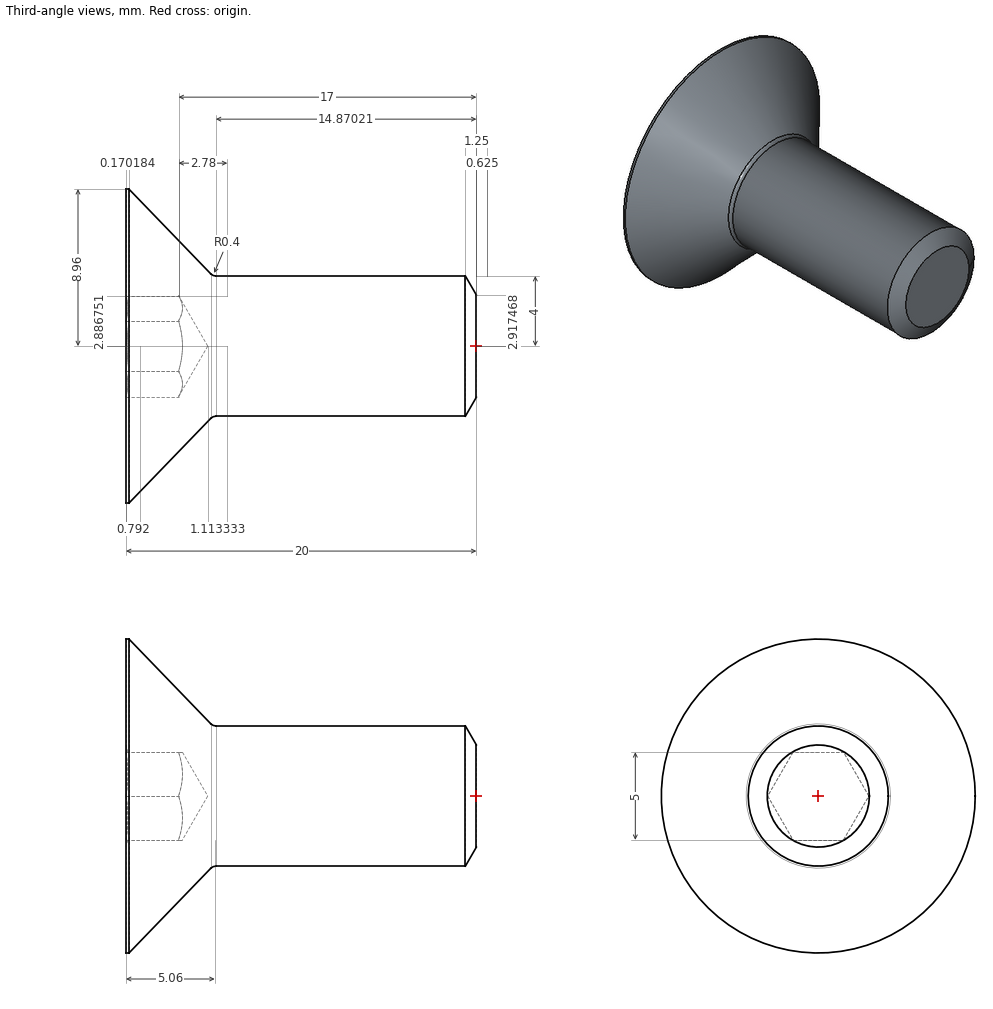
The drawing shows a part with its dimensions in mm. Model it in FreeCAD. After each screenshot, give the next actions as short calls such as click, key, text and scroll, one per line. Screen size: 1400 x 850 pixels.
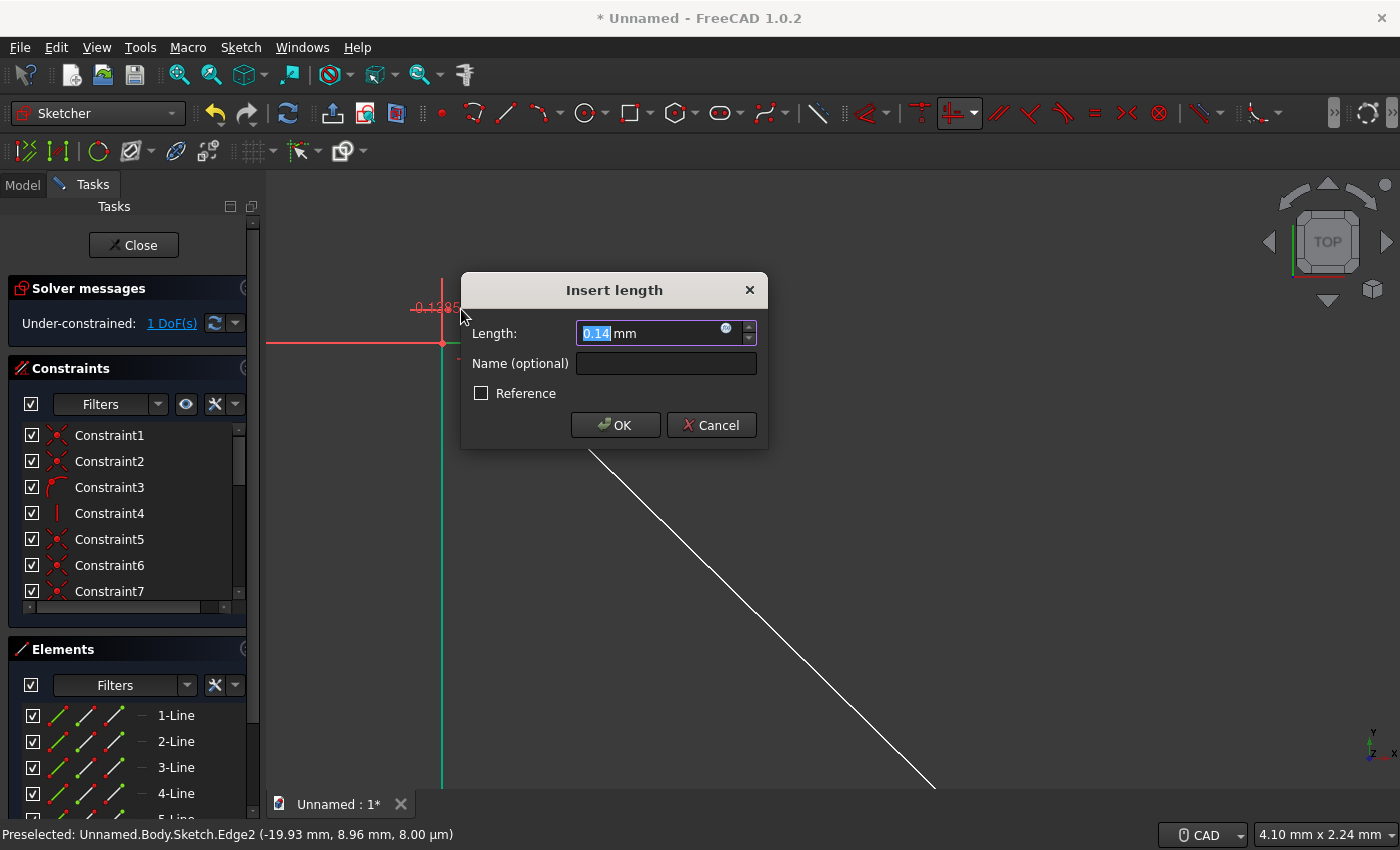
text(0.170184)
key(Return)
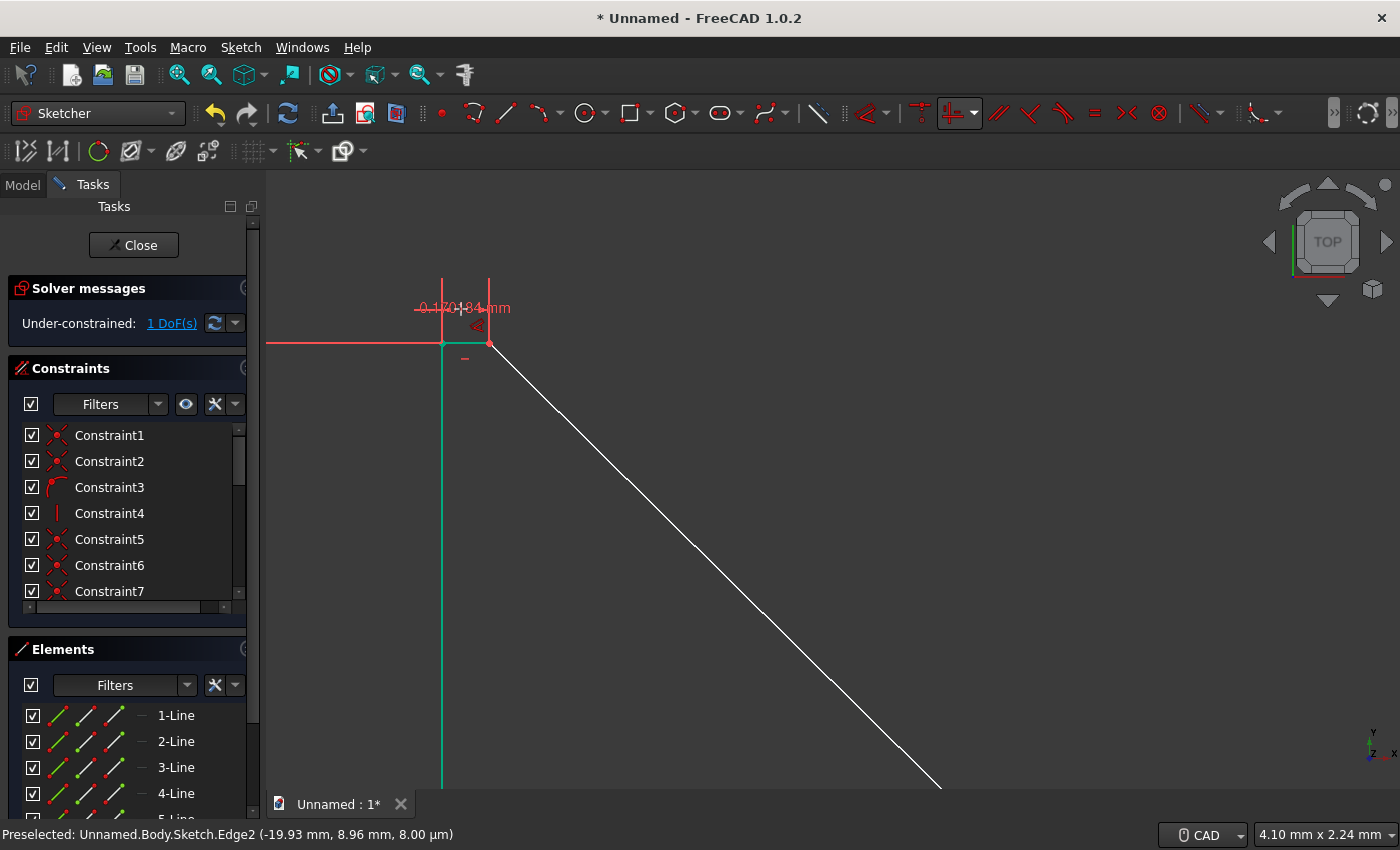
scroll(460, 342, down, 11)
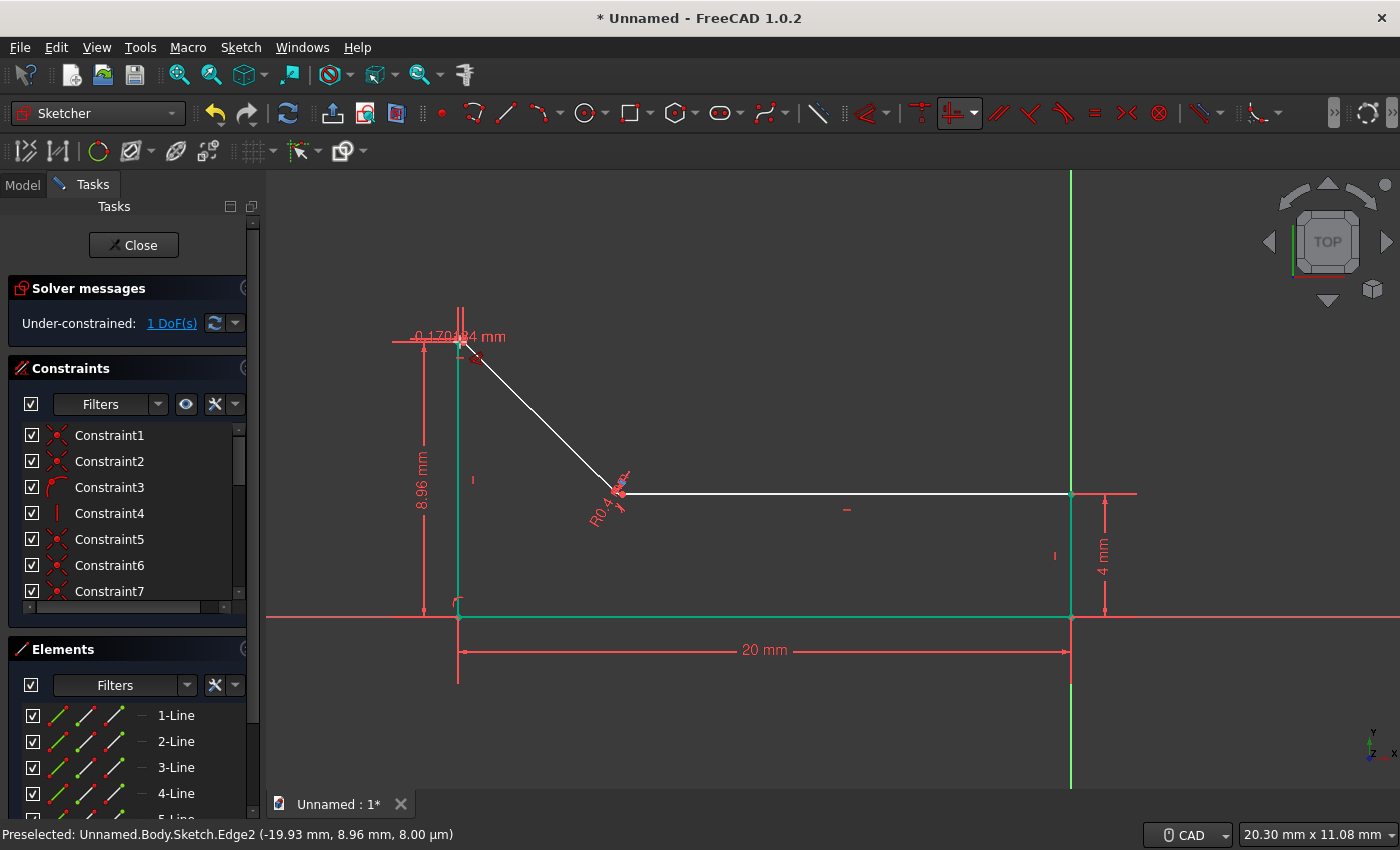
click(937, 494)
click(847, 528)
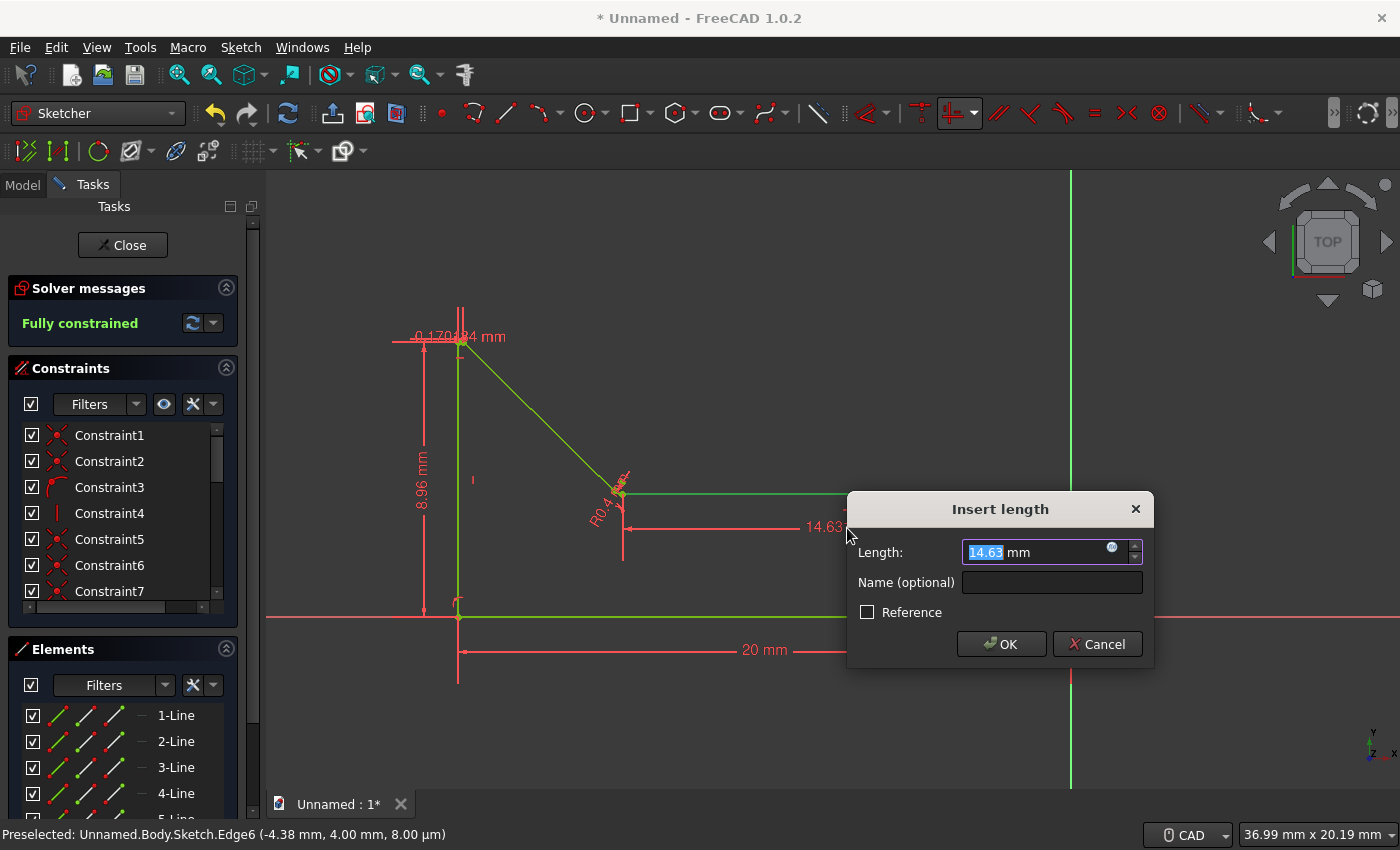
text(14.87021)
key(Return)
key(Escape)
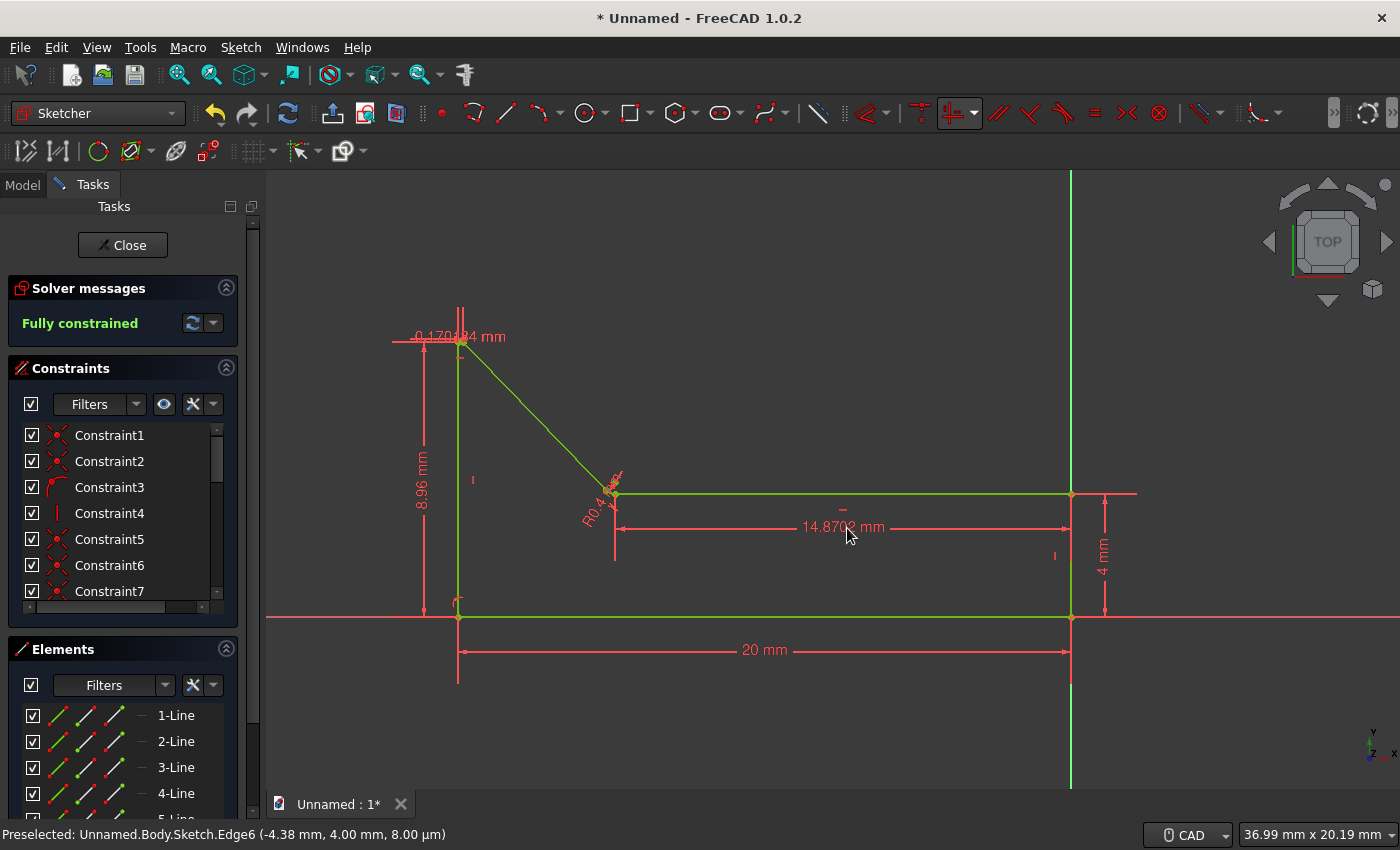
click(123, 245)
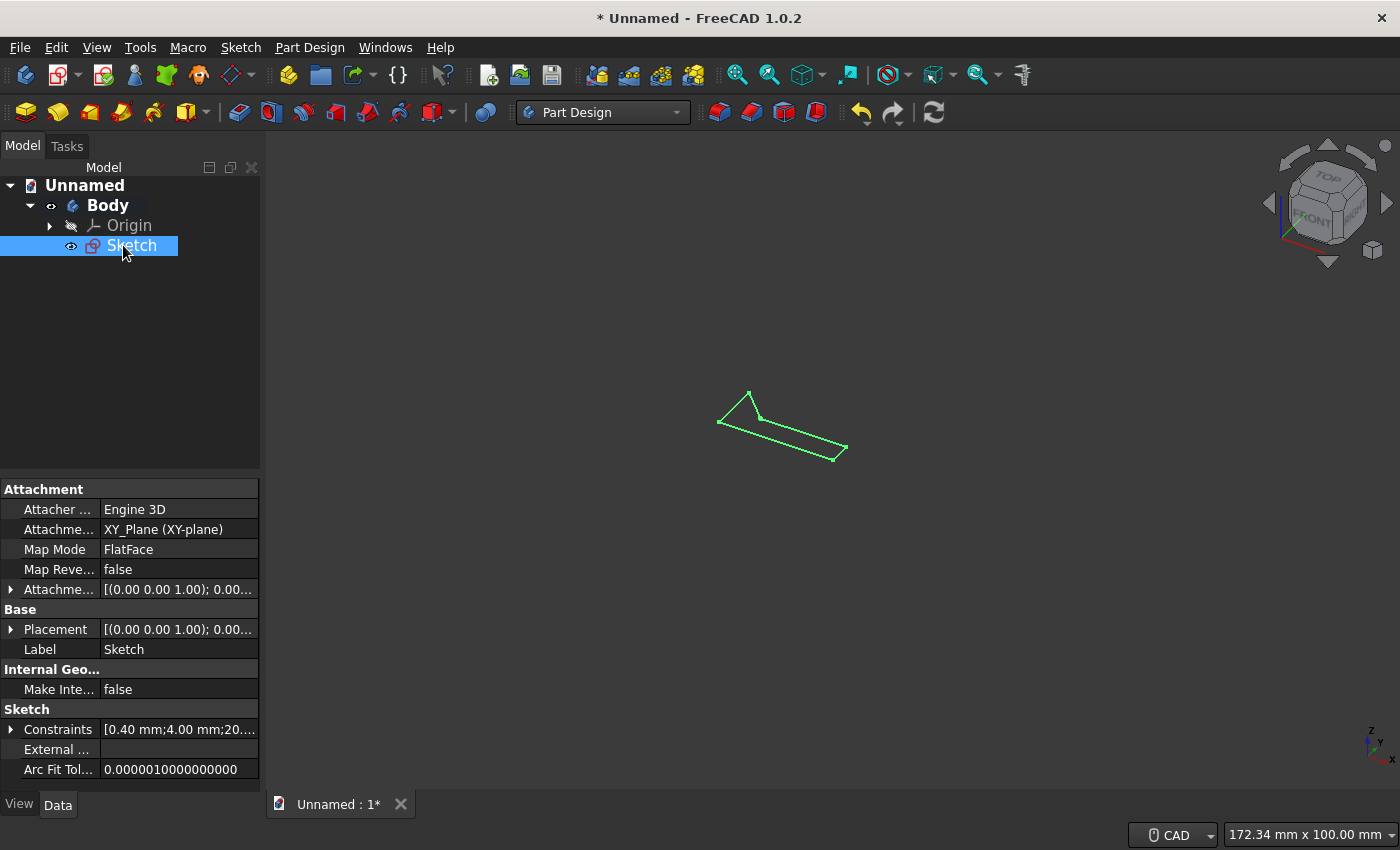
click(58, 112)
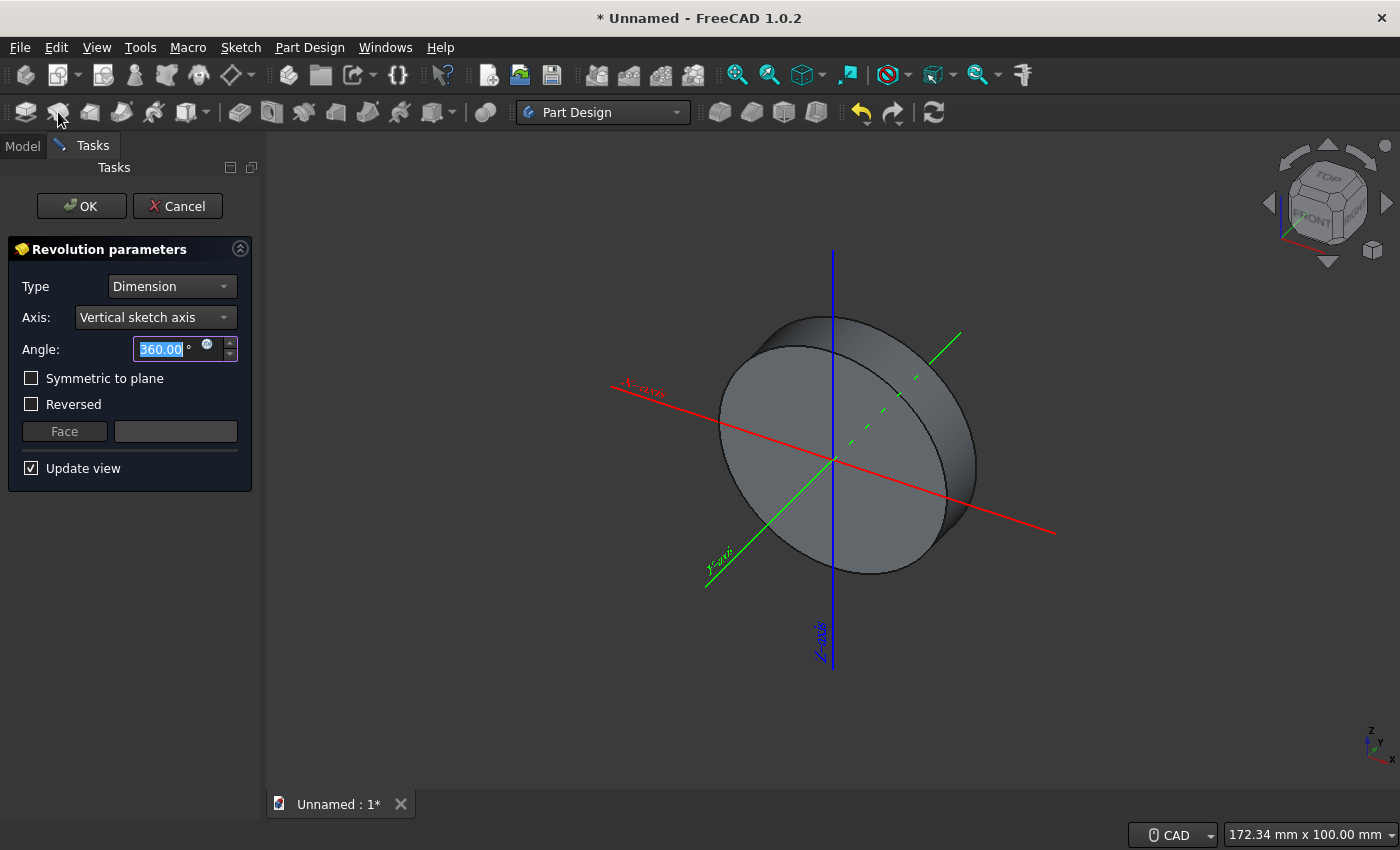
click(156, 318)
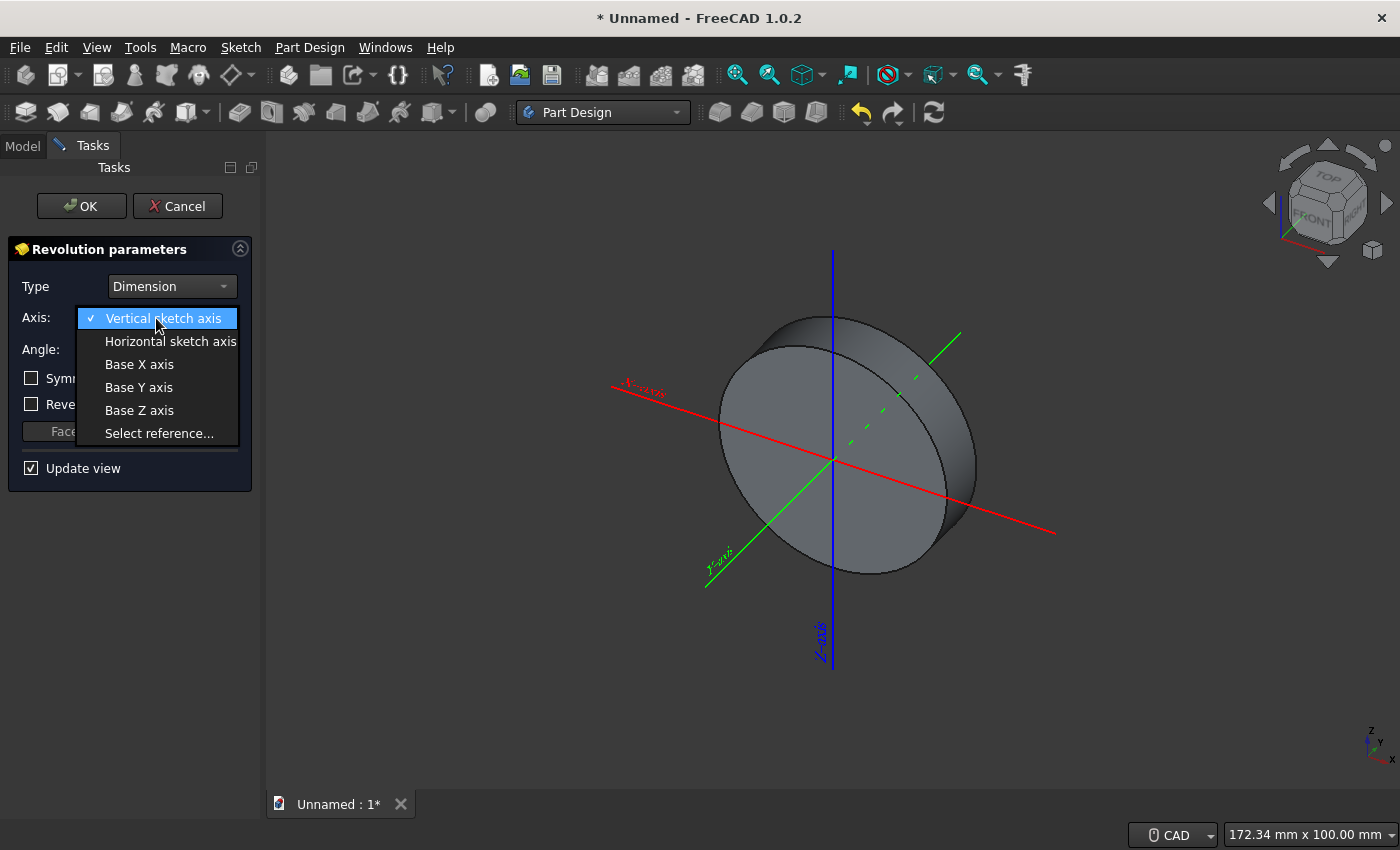
click(156, 342)